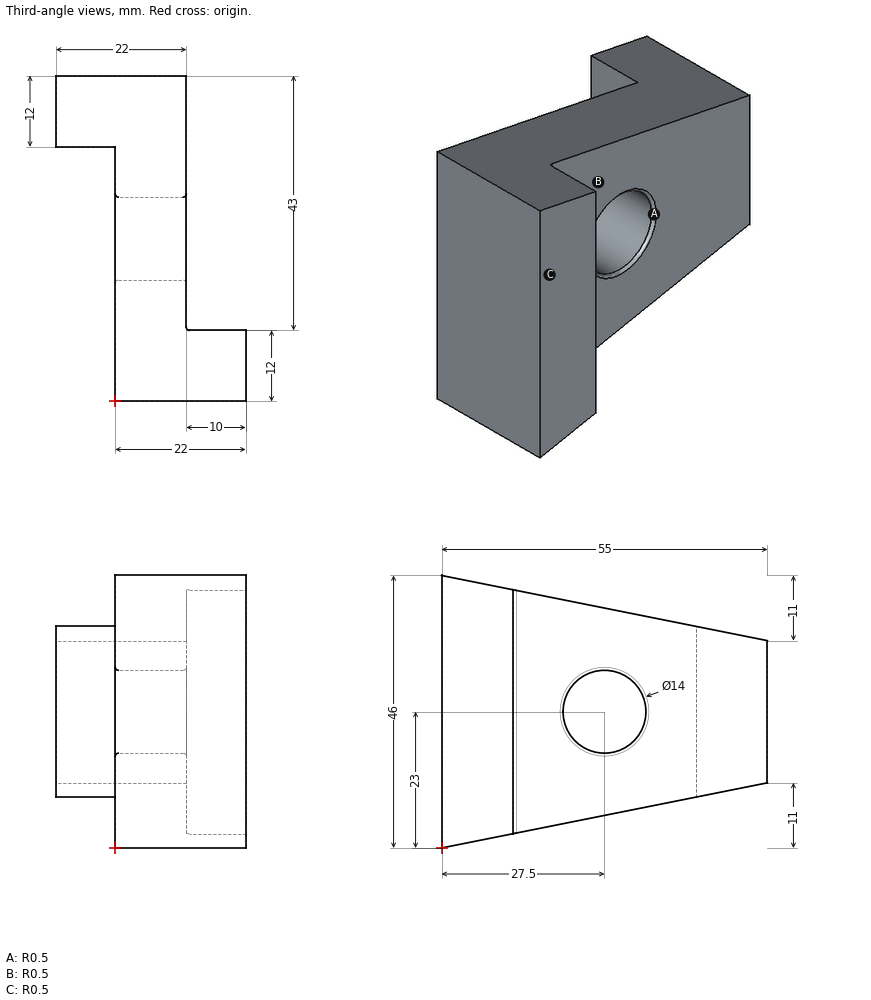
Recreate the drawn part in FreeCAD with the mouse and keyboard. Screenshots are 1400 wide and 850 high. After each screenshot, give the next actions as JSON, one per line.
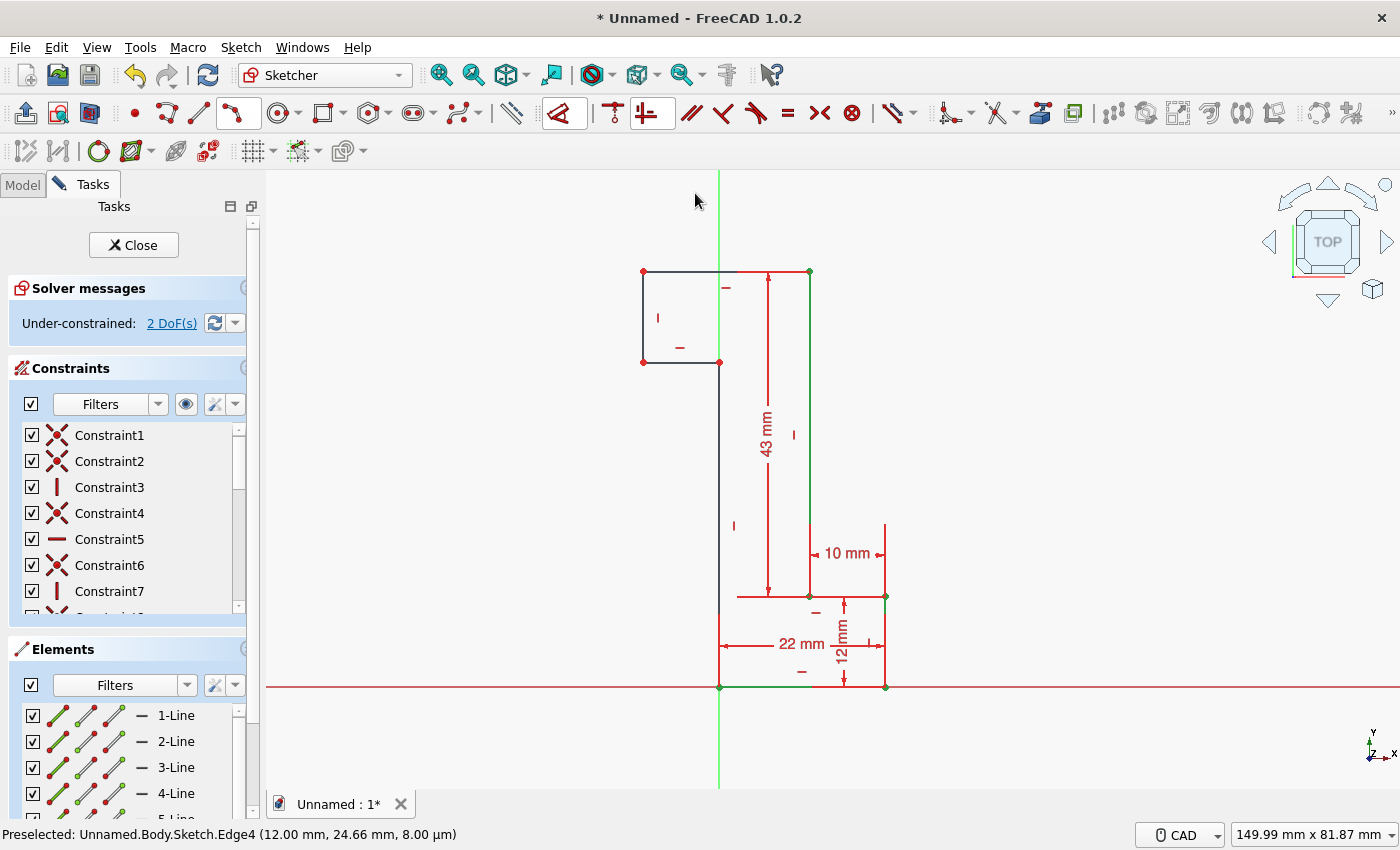
{"action": "left_click", "coordinate": [760, 272]}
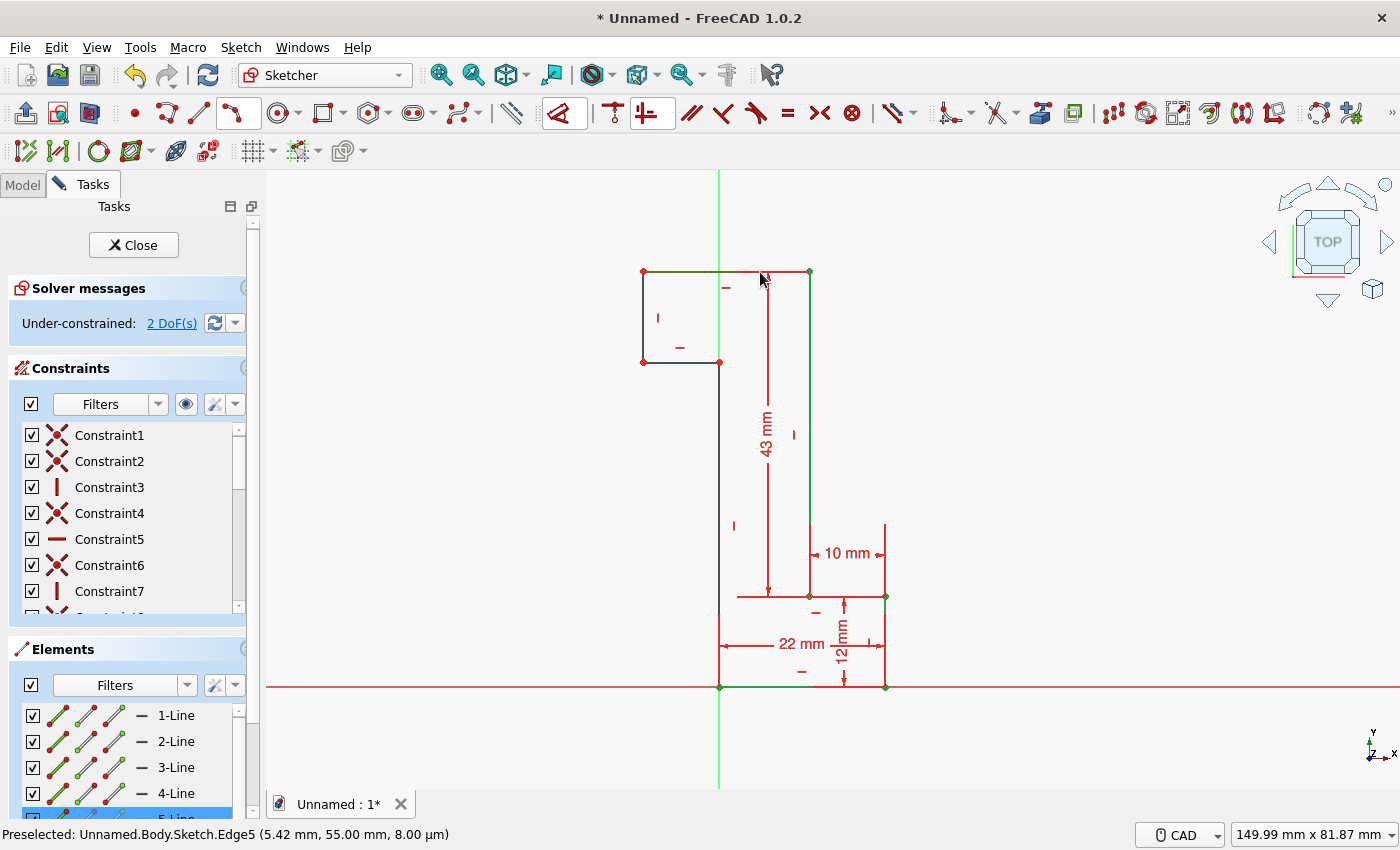
{"action": "left_click", "coordinate": [582, 114]}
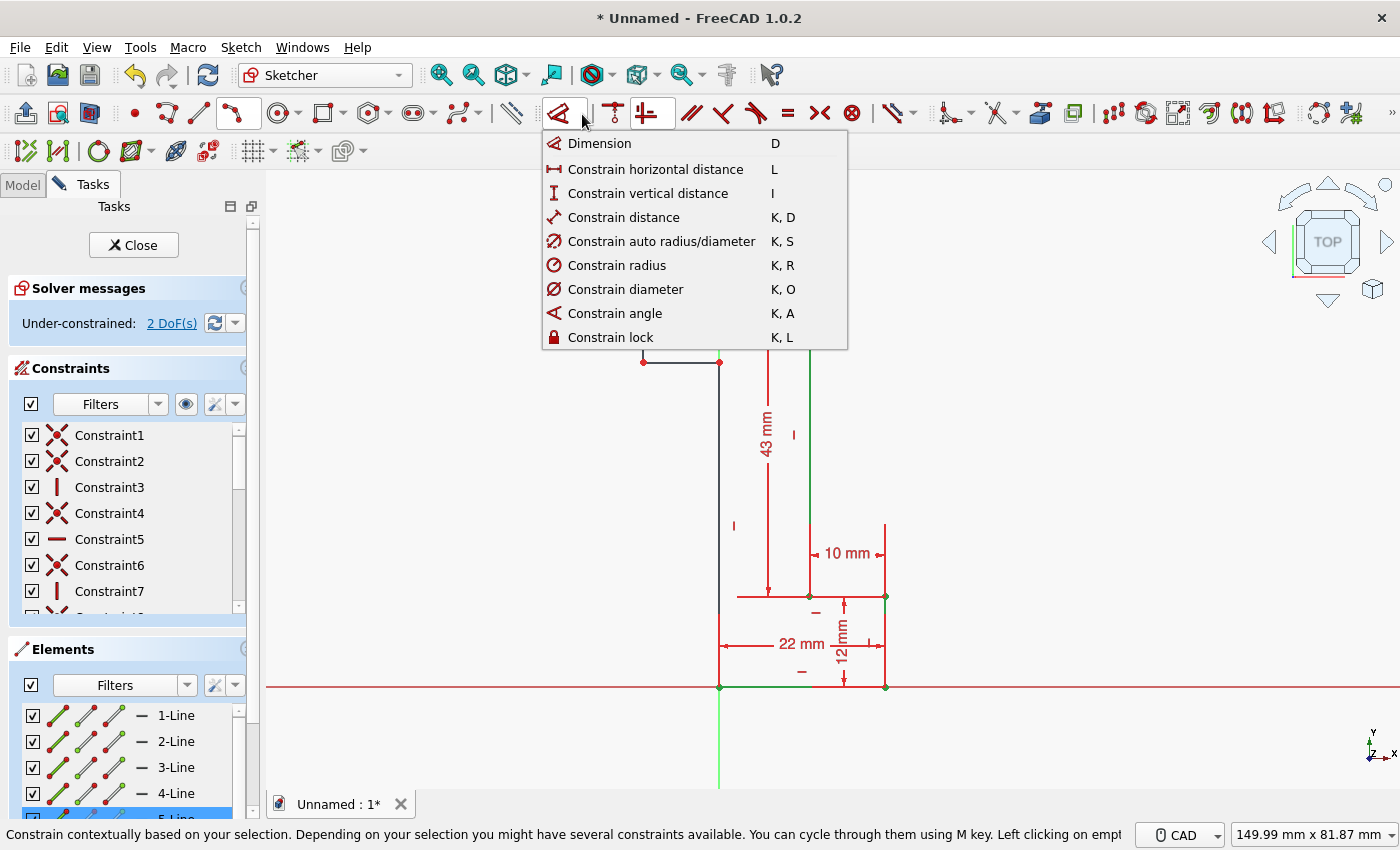
{"action": "left_click", "coordinate": [695, 169]}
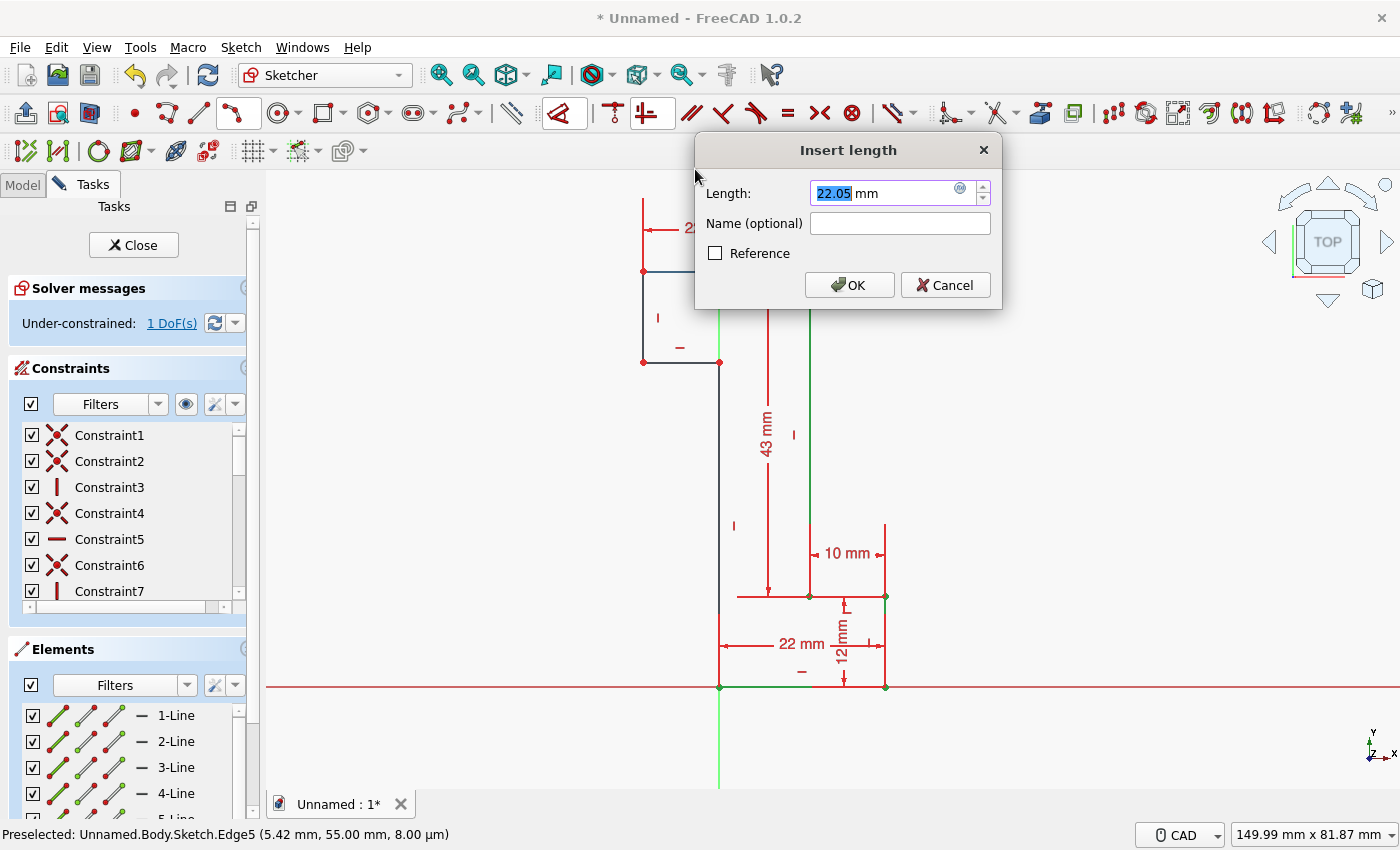
{"action": "type", "text": "22"}
{"action": "key", "text": "Return"}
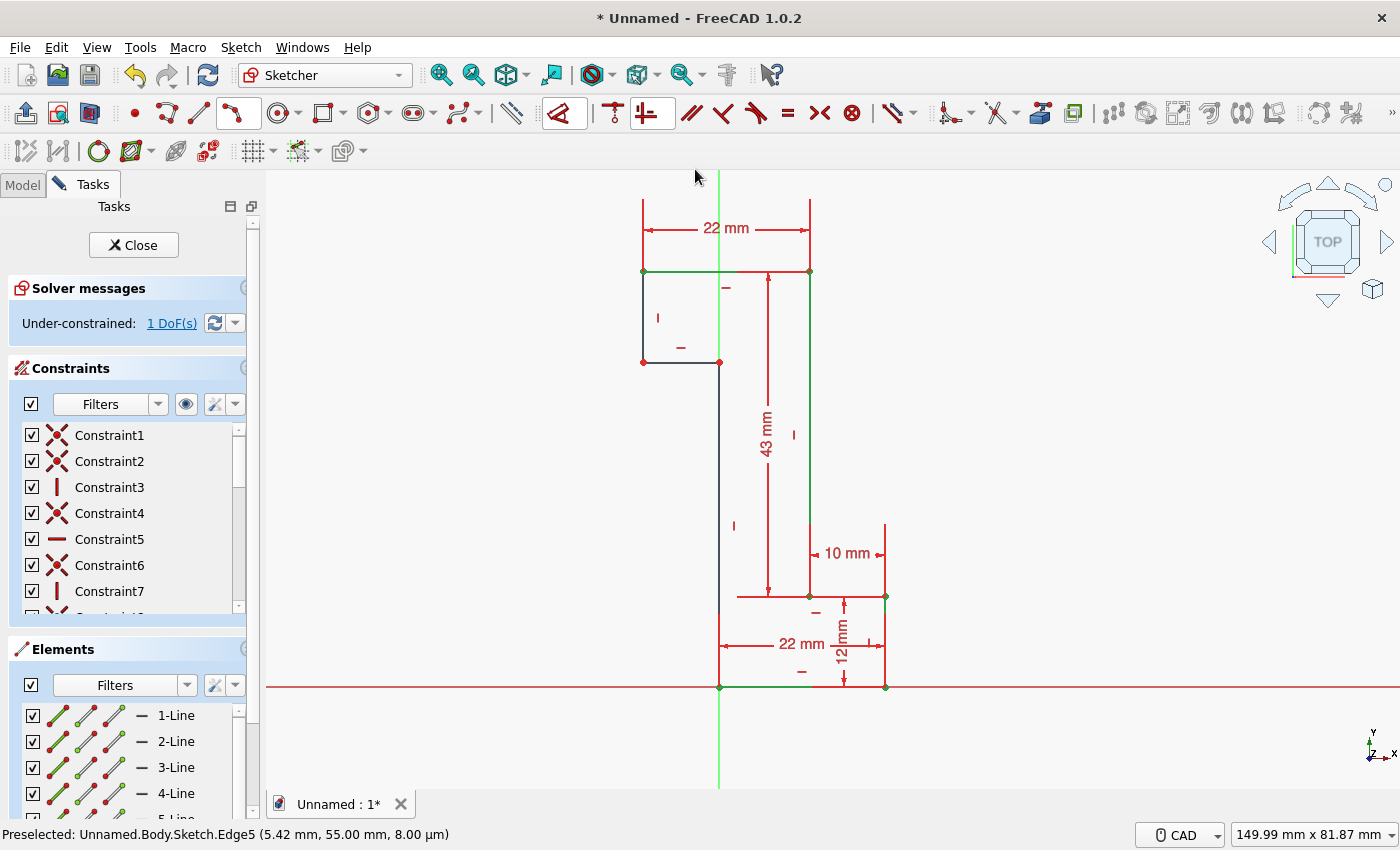
{"action": "left_click", "coordinate": [643, 299]}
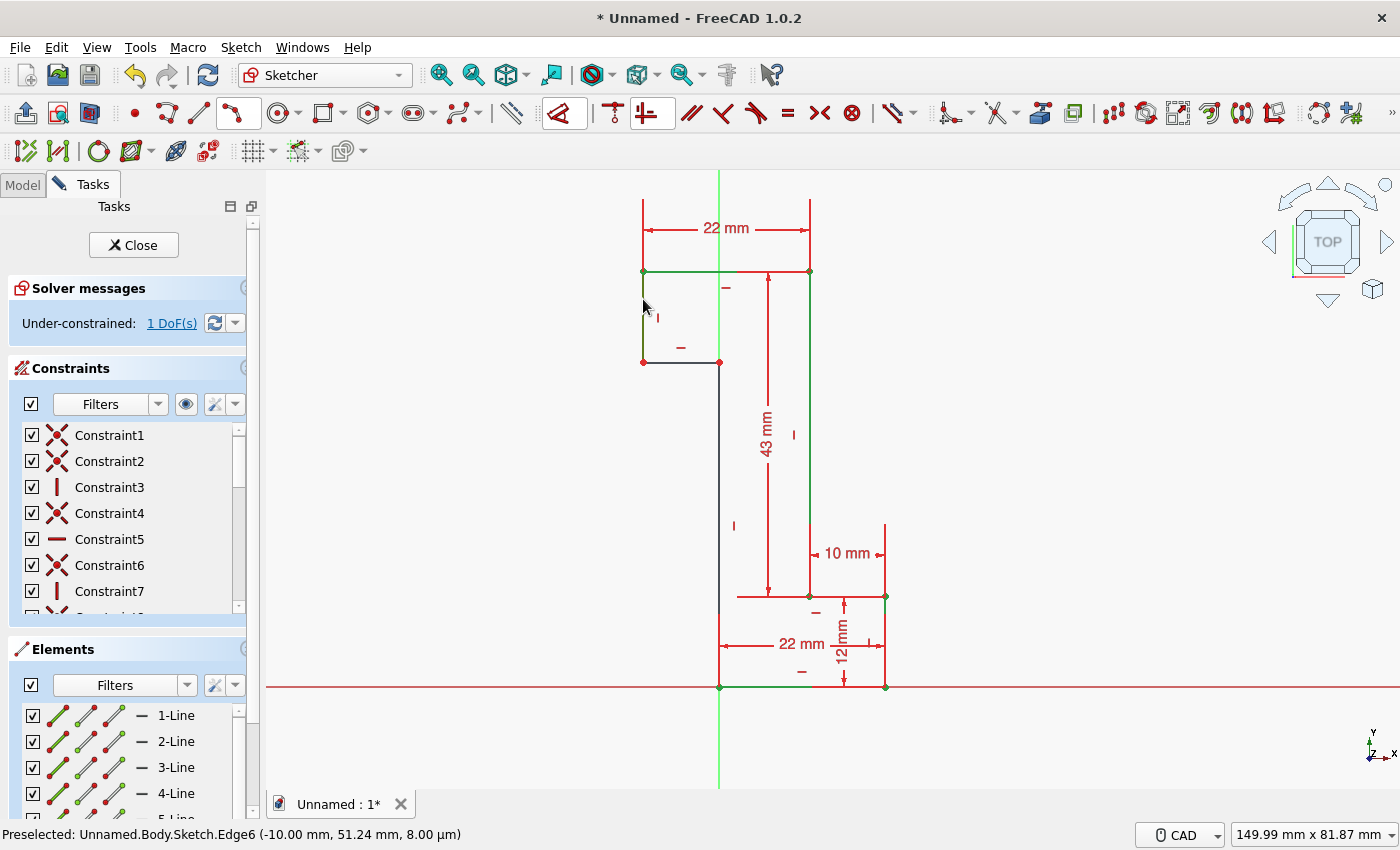
{"action": "key", "text": "i"}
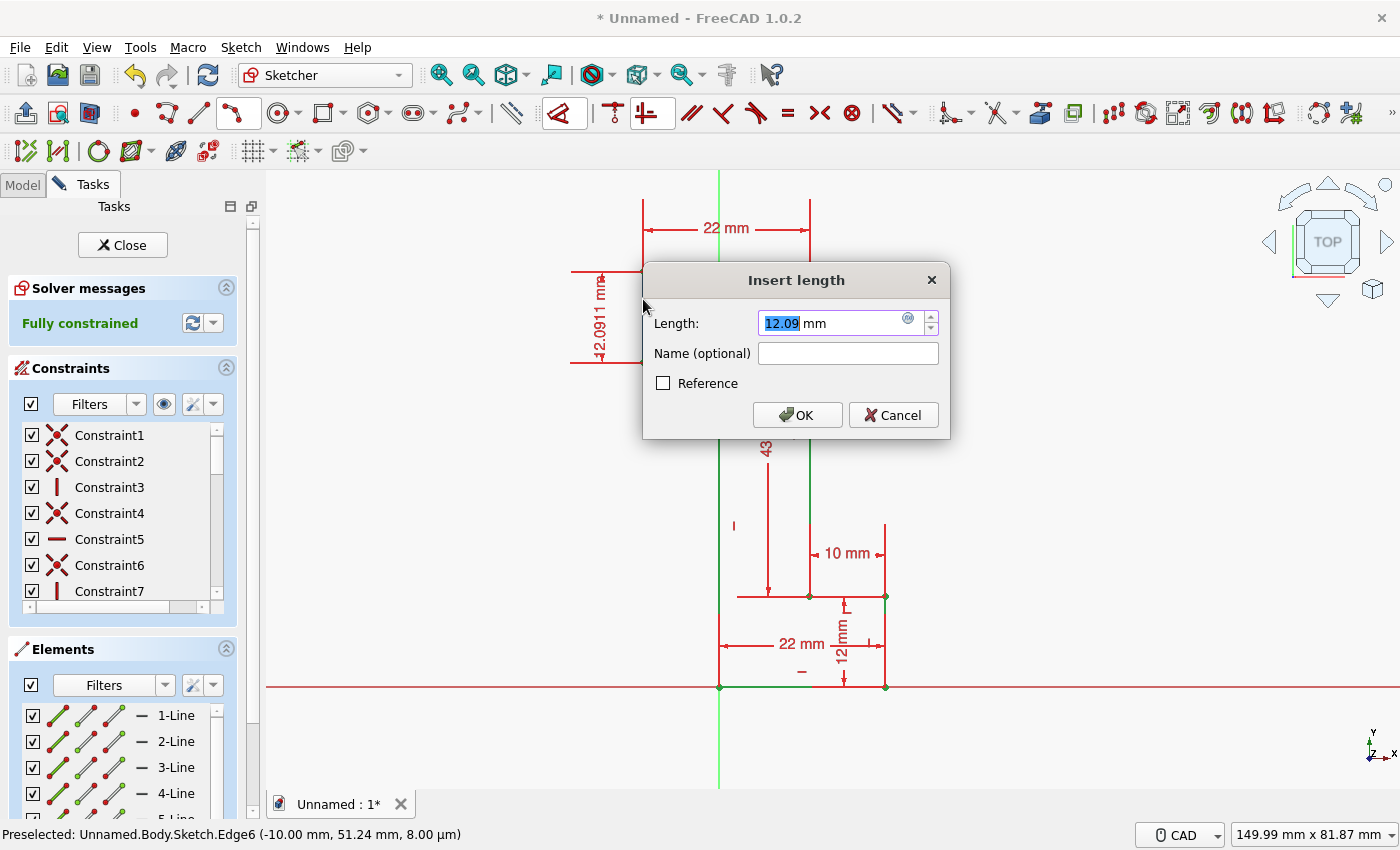
{"action": "type", "text": "12"}
{"action": "key", "text": "Return"}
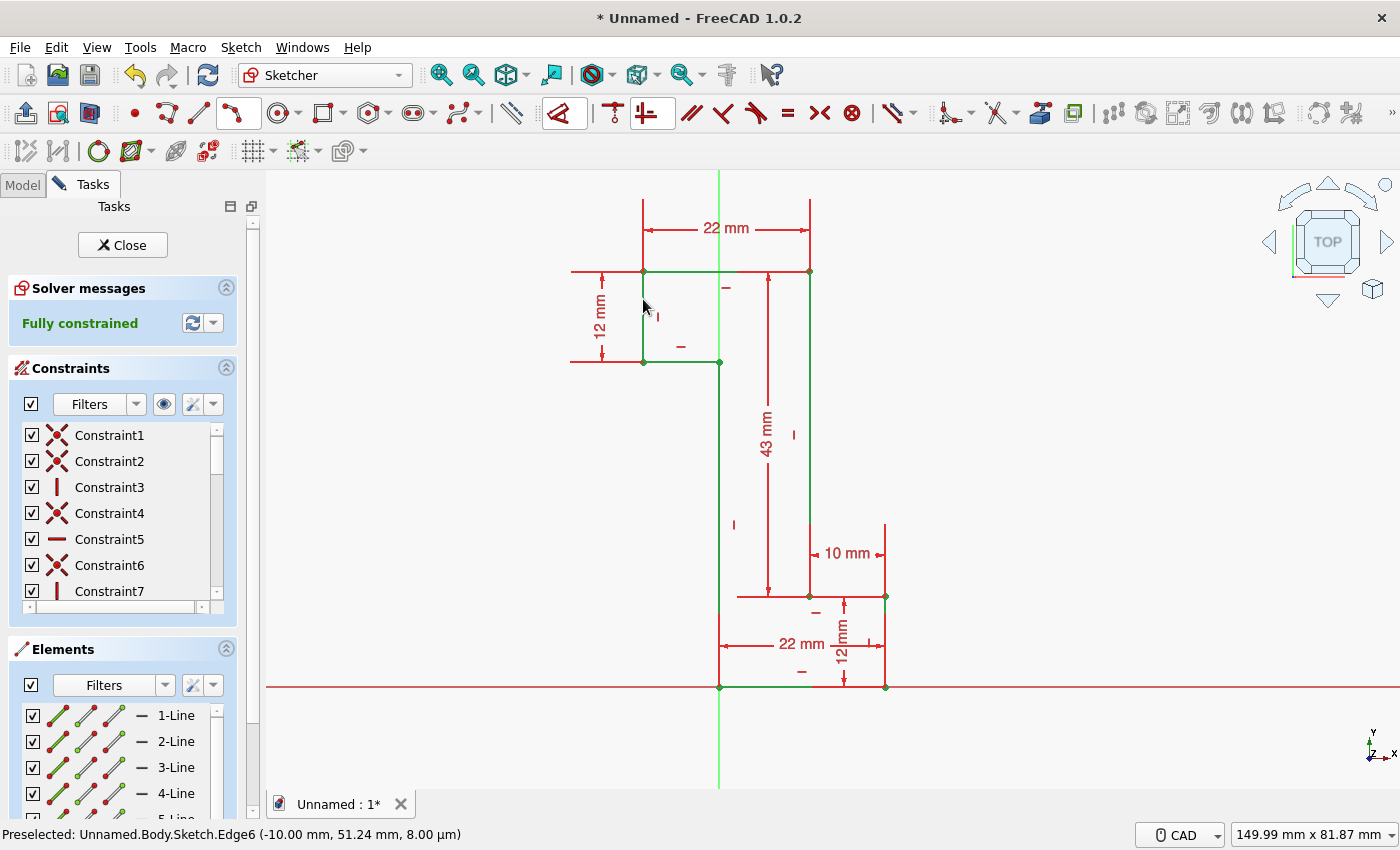
{"action": "left_click", "coordinate": [123, 245]}